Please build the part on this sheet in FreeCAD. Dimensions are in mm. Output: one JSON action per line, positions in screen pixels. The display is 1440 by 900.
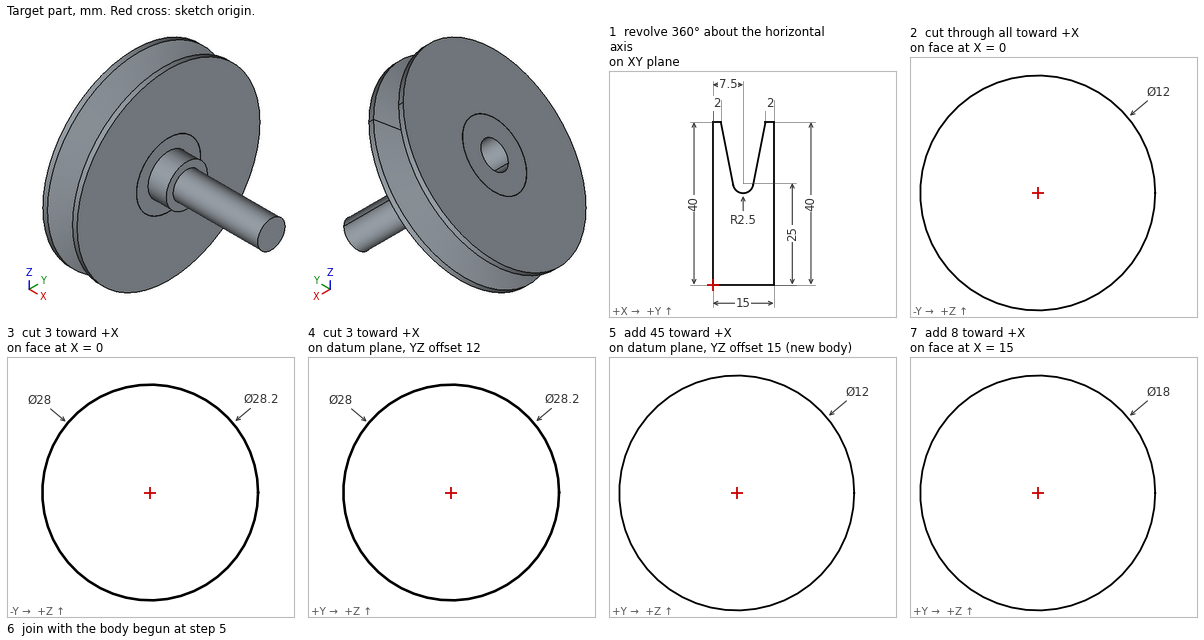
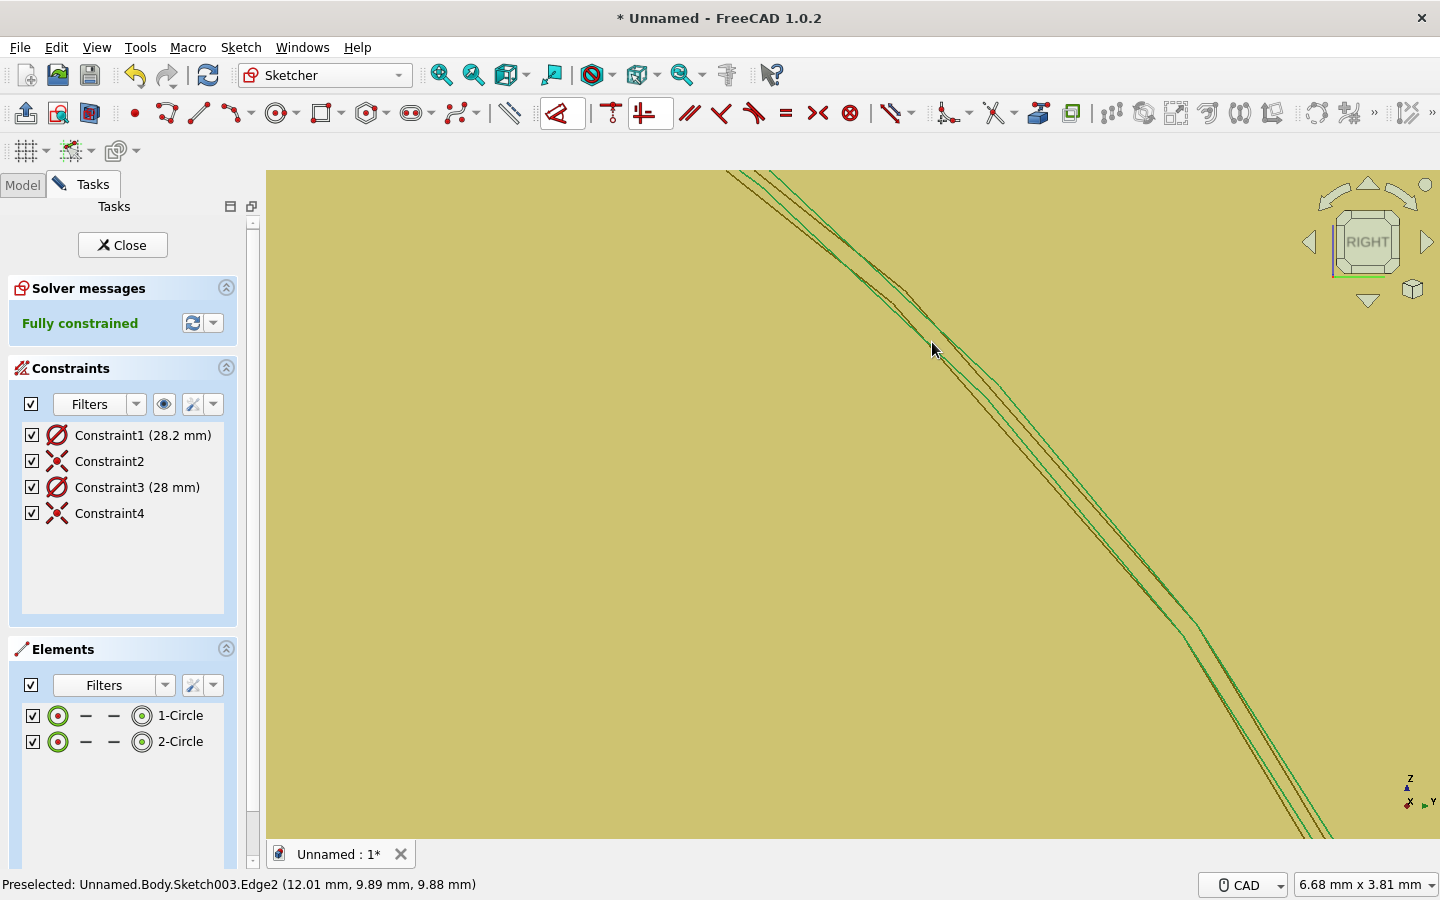
{"action": "left_click", "coordinate": [123, 245]}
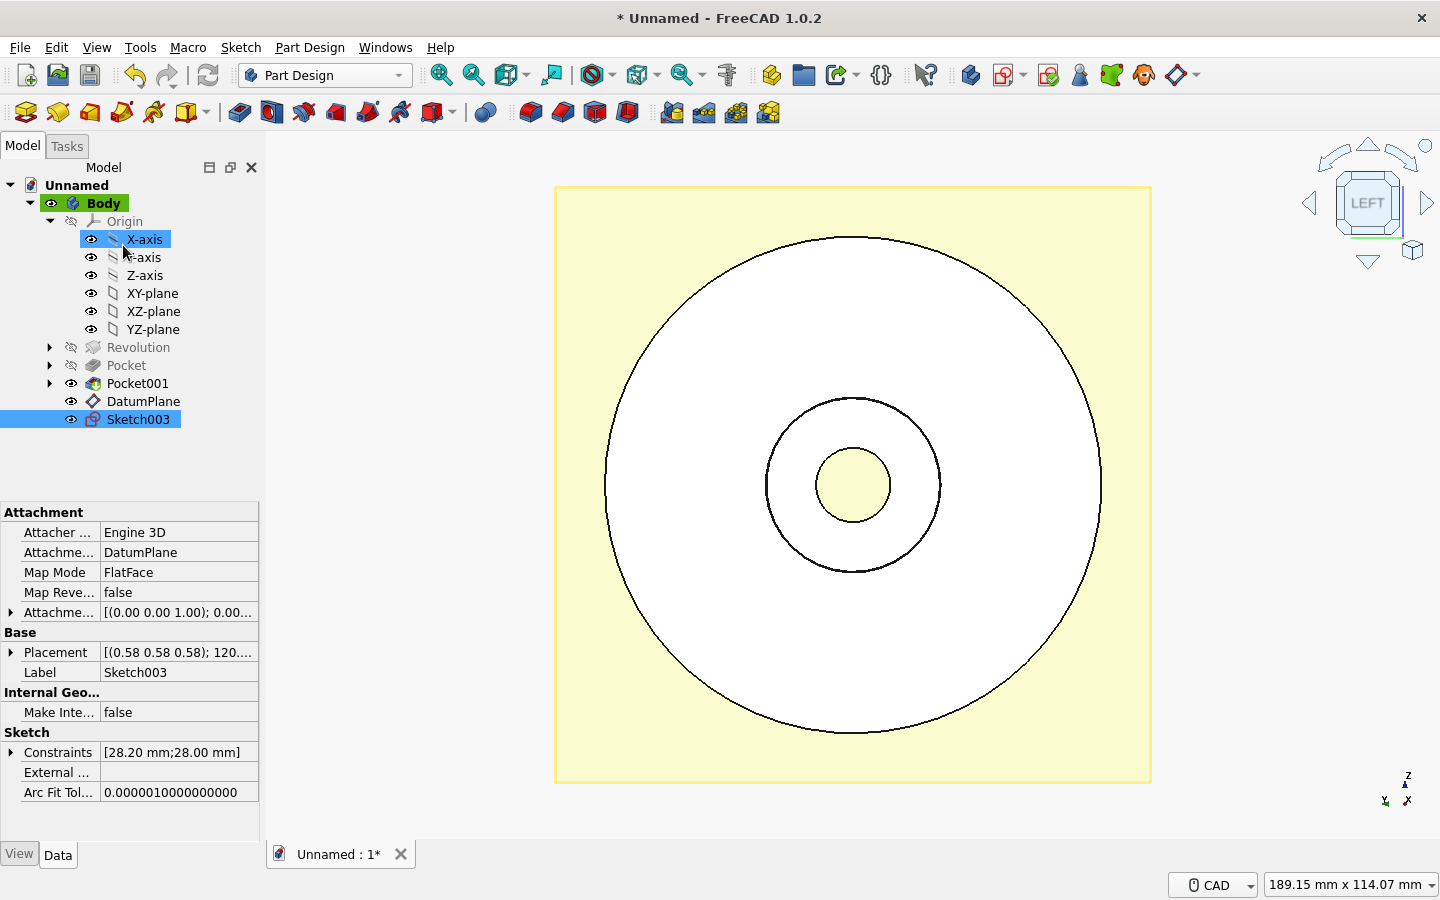
{"action": "left_click", "coordinate": [240, 112]}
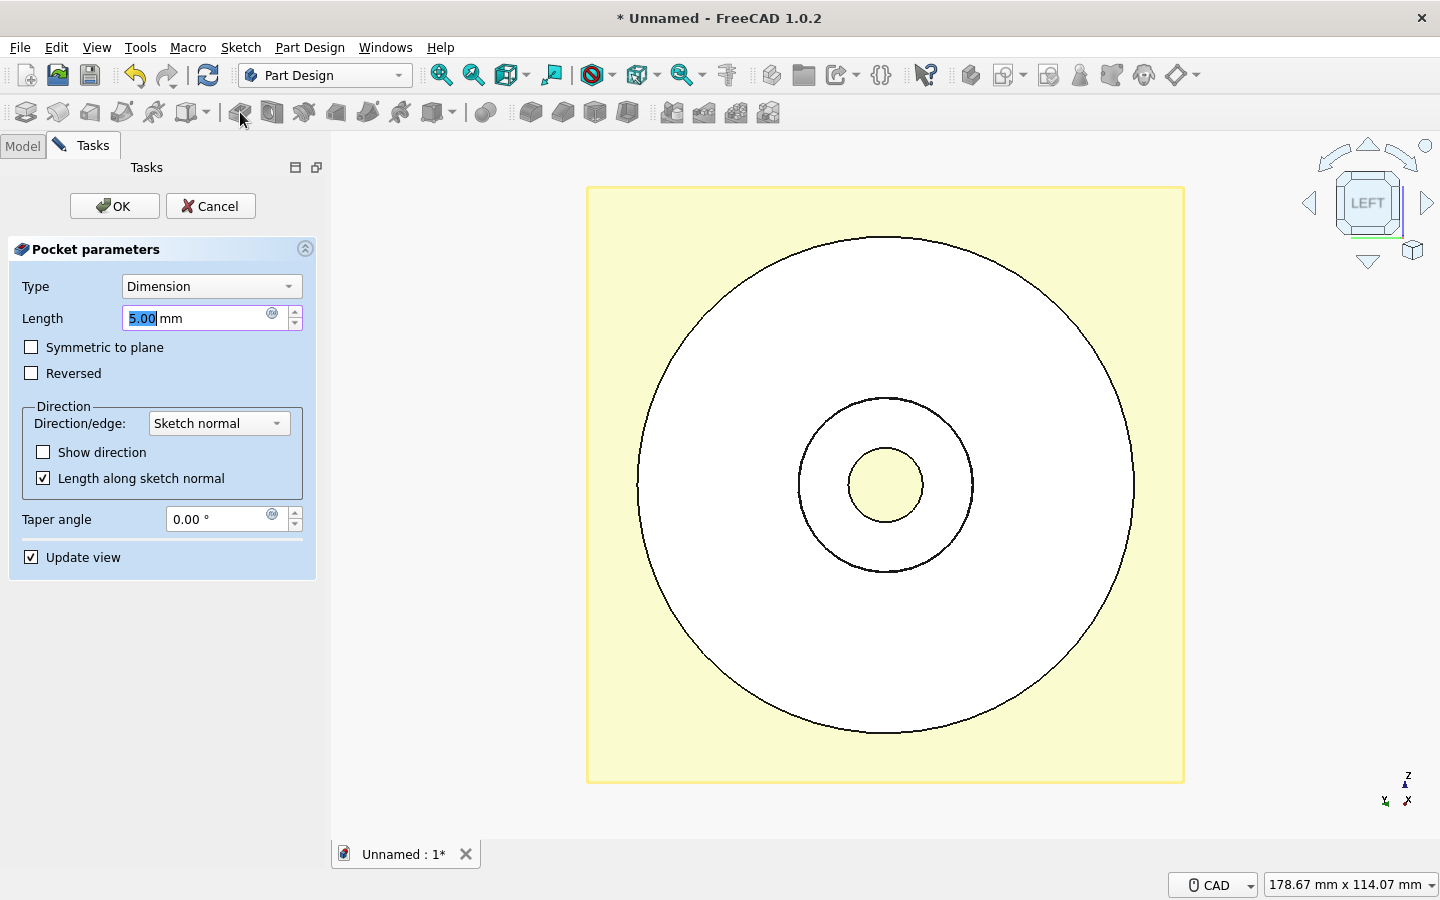
{"action": "type", "text": "3"}
{"action": "key", "text": "Tab"}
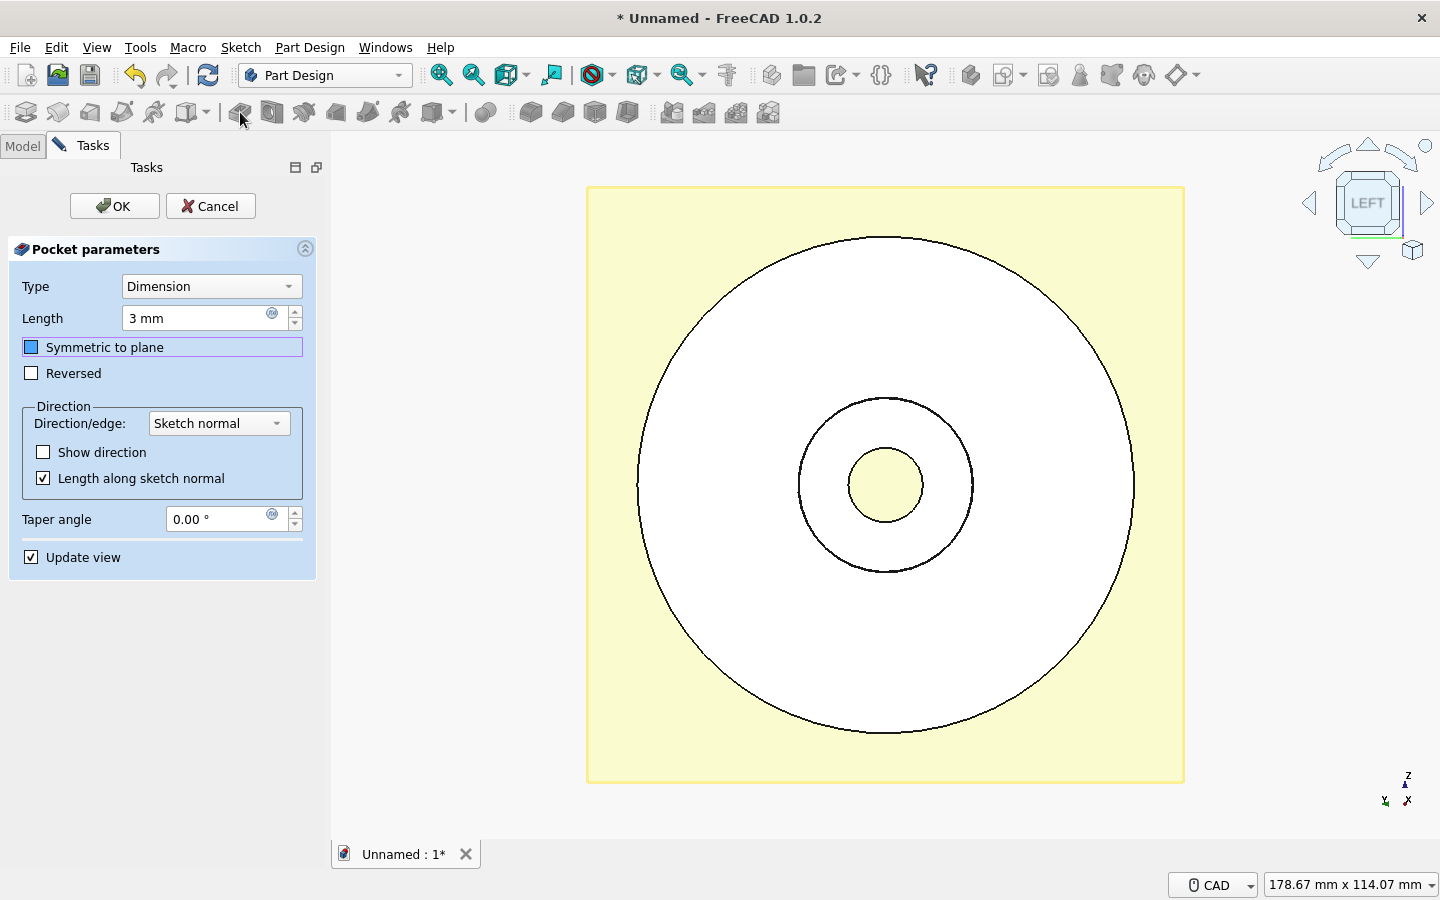
{"action": "left_click", "coordinate": [30, 373]}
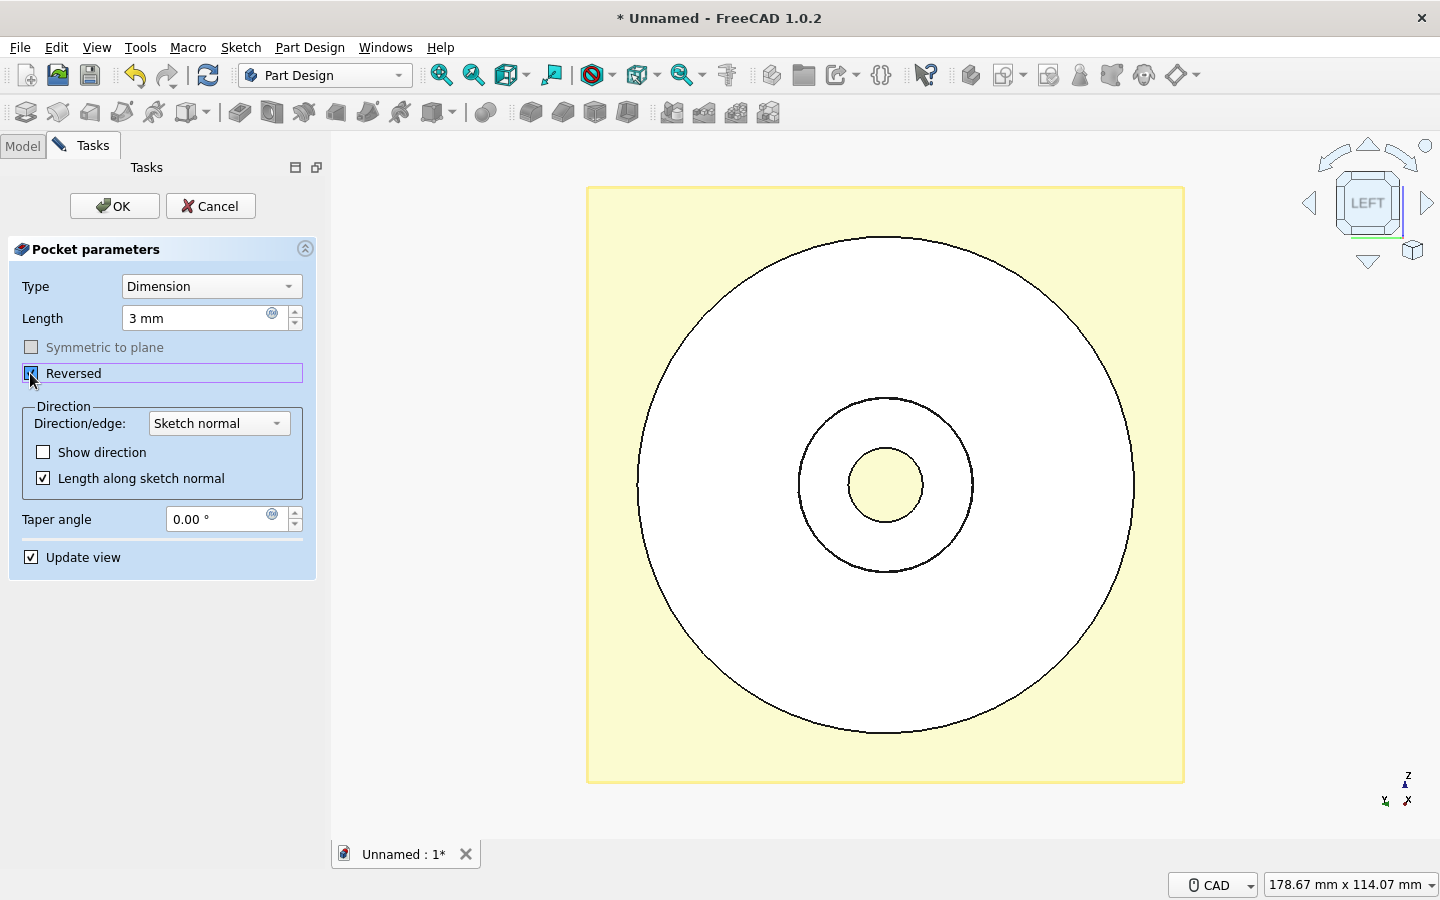
{"action": "left_click", "coordinate": [115, 206]}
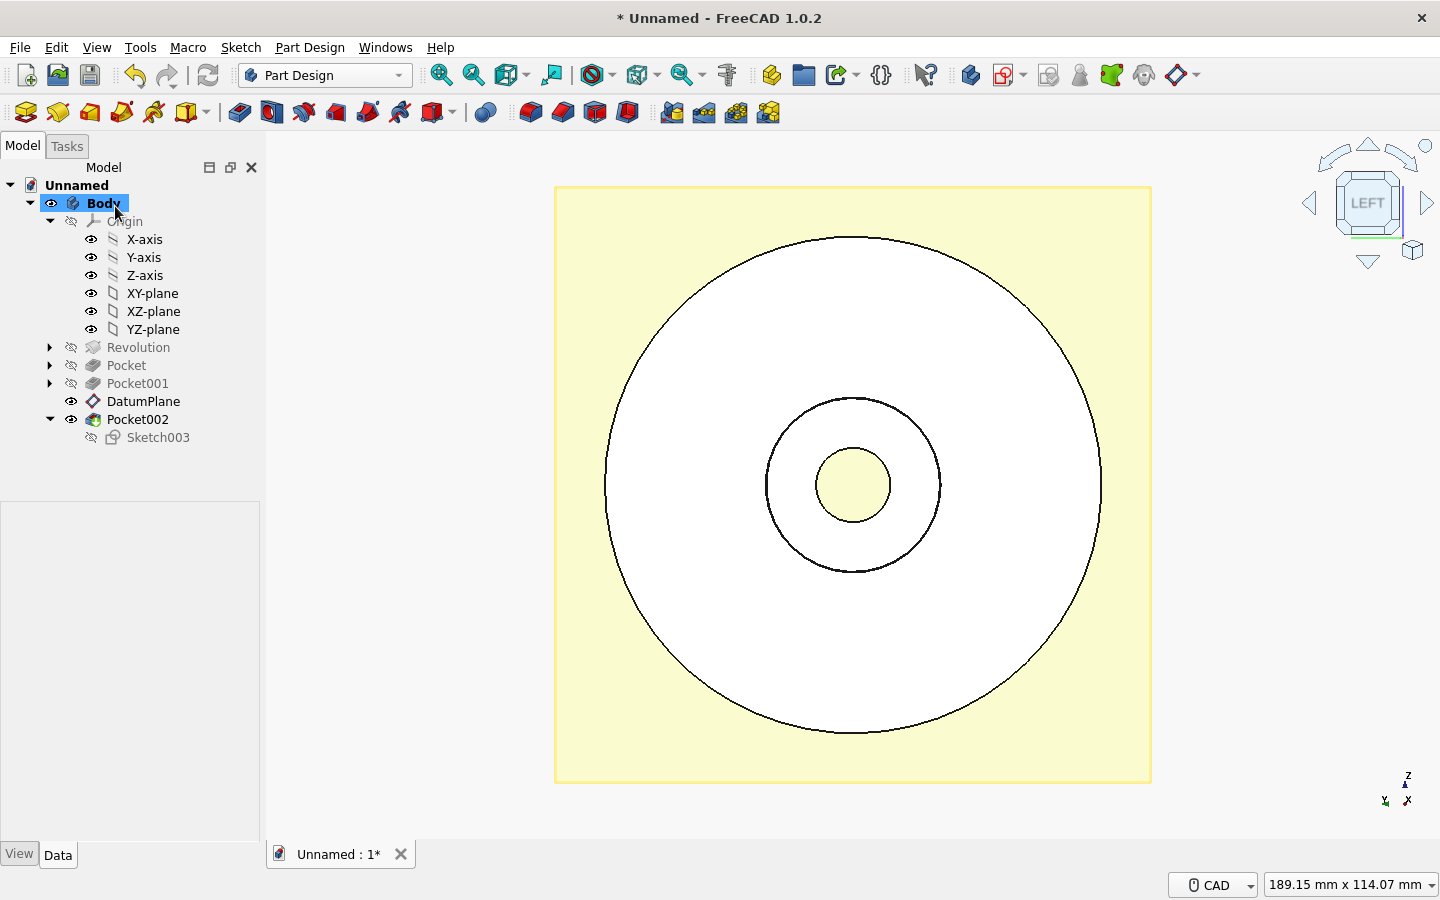
{"action": "left_click", "coordinate": [116, 401]}
{"action": "key", "text": "space"}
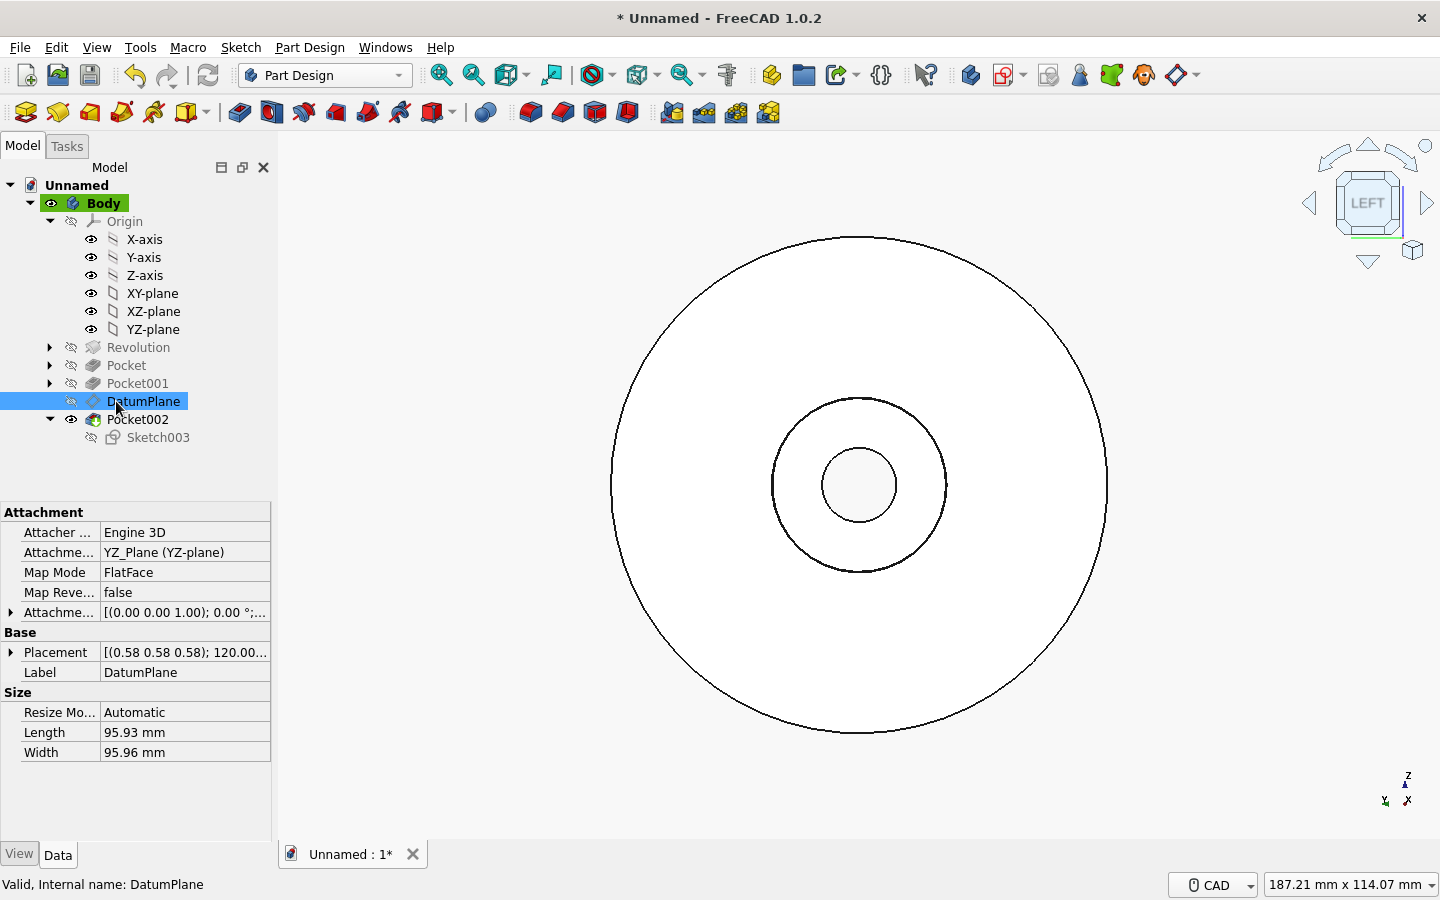
{"action": "left_click", "coordinate": [318, 799]}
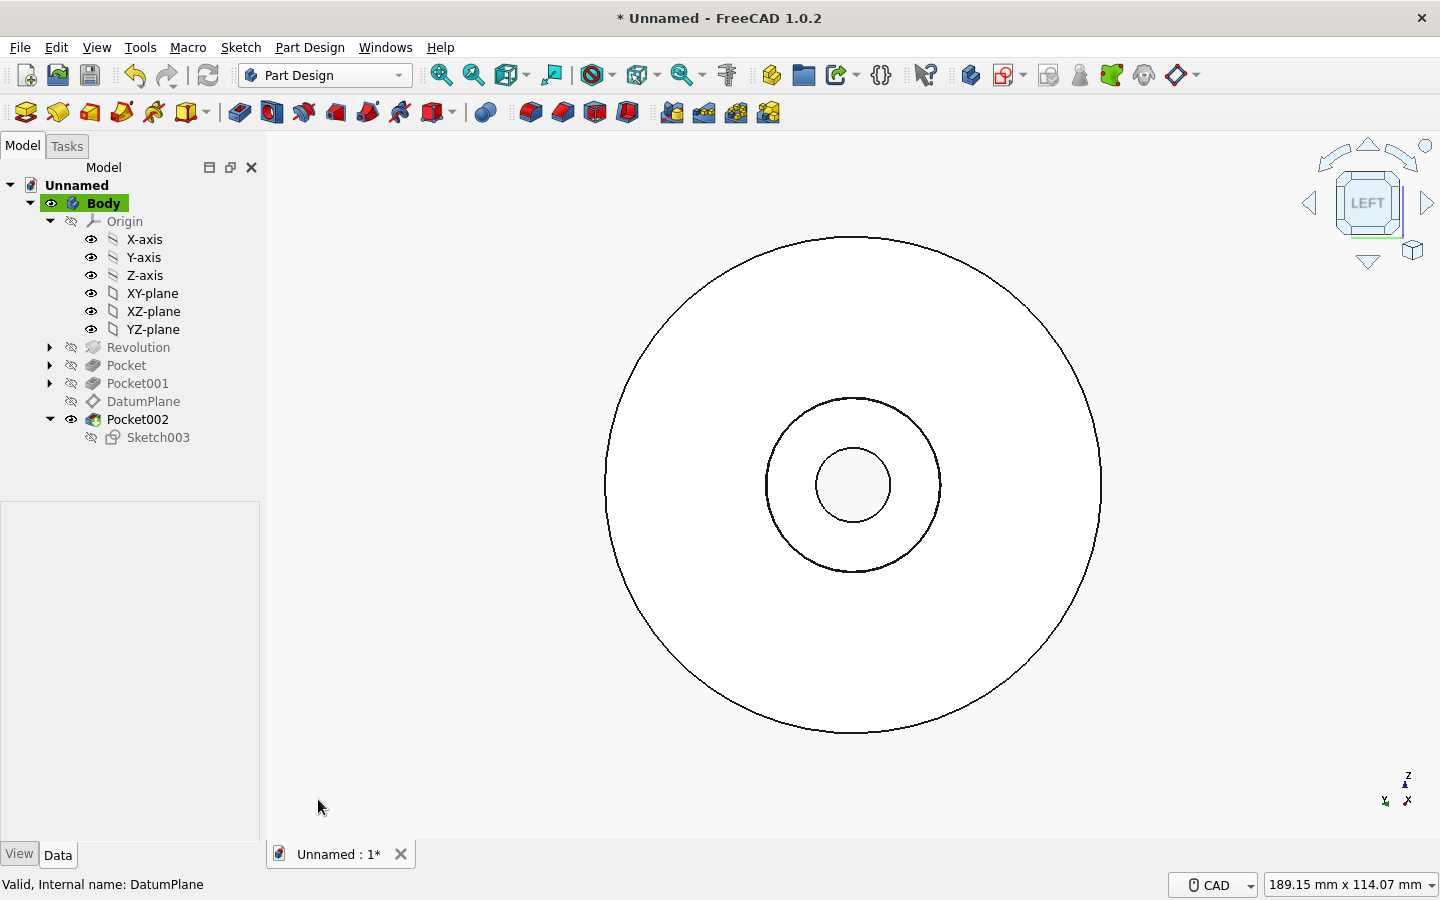
{"action": "left_click", "coordinate": [972, 76]}